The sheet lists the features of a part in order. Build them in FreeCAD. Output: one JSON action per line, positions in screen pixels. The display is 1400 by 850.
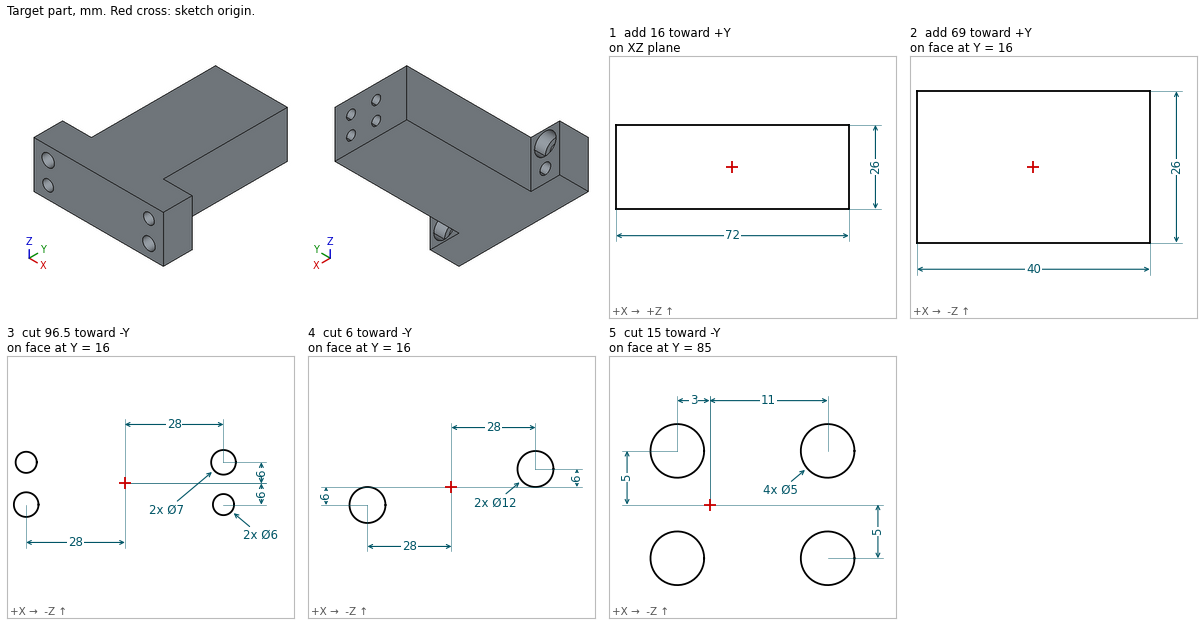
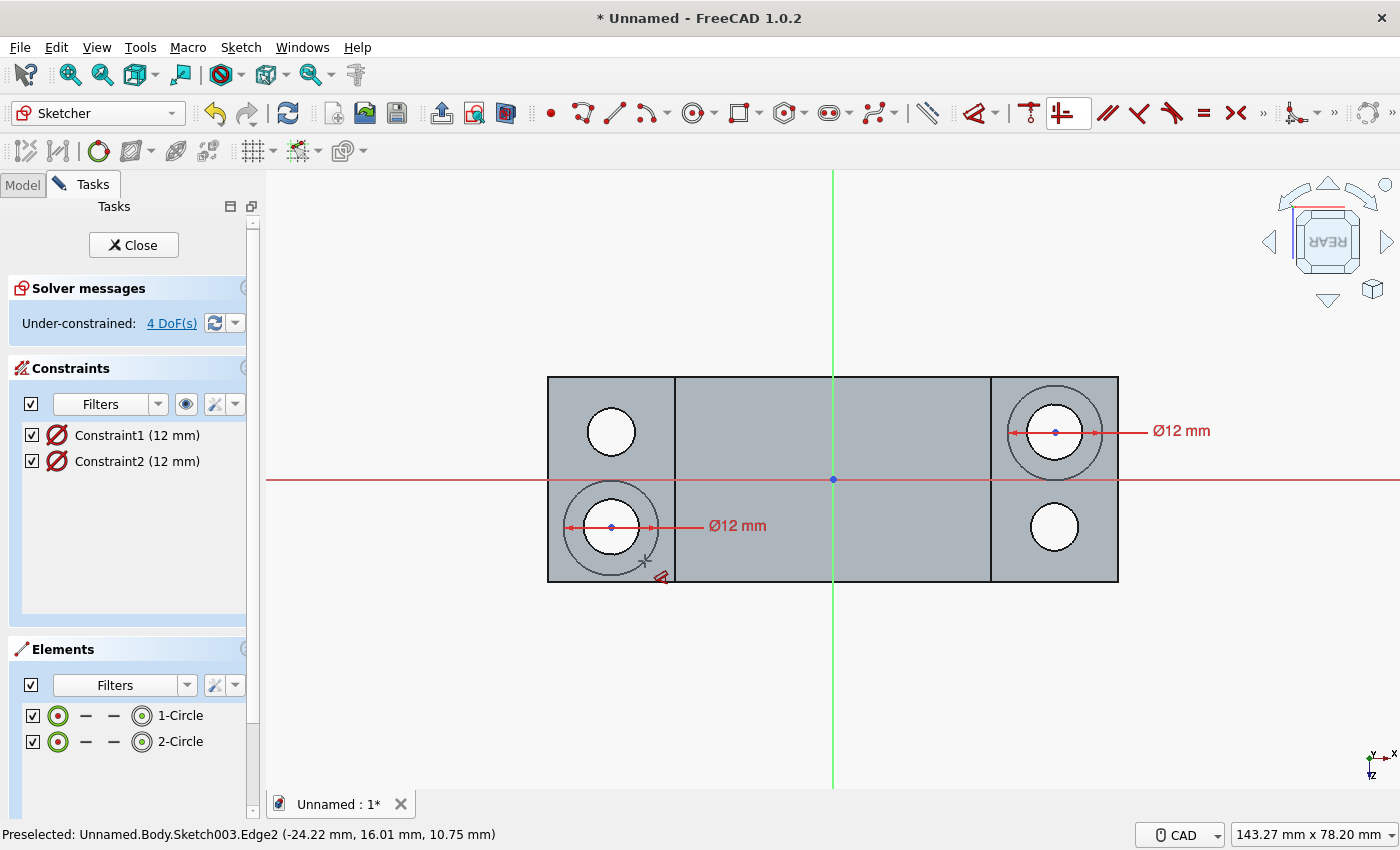
{"action": "left_click", "coordinate": [1055, 433]}
{"action": "left_click", "coordinate": [799, 456]}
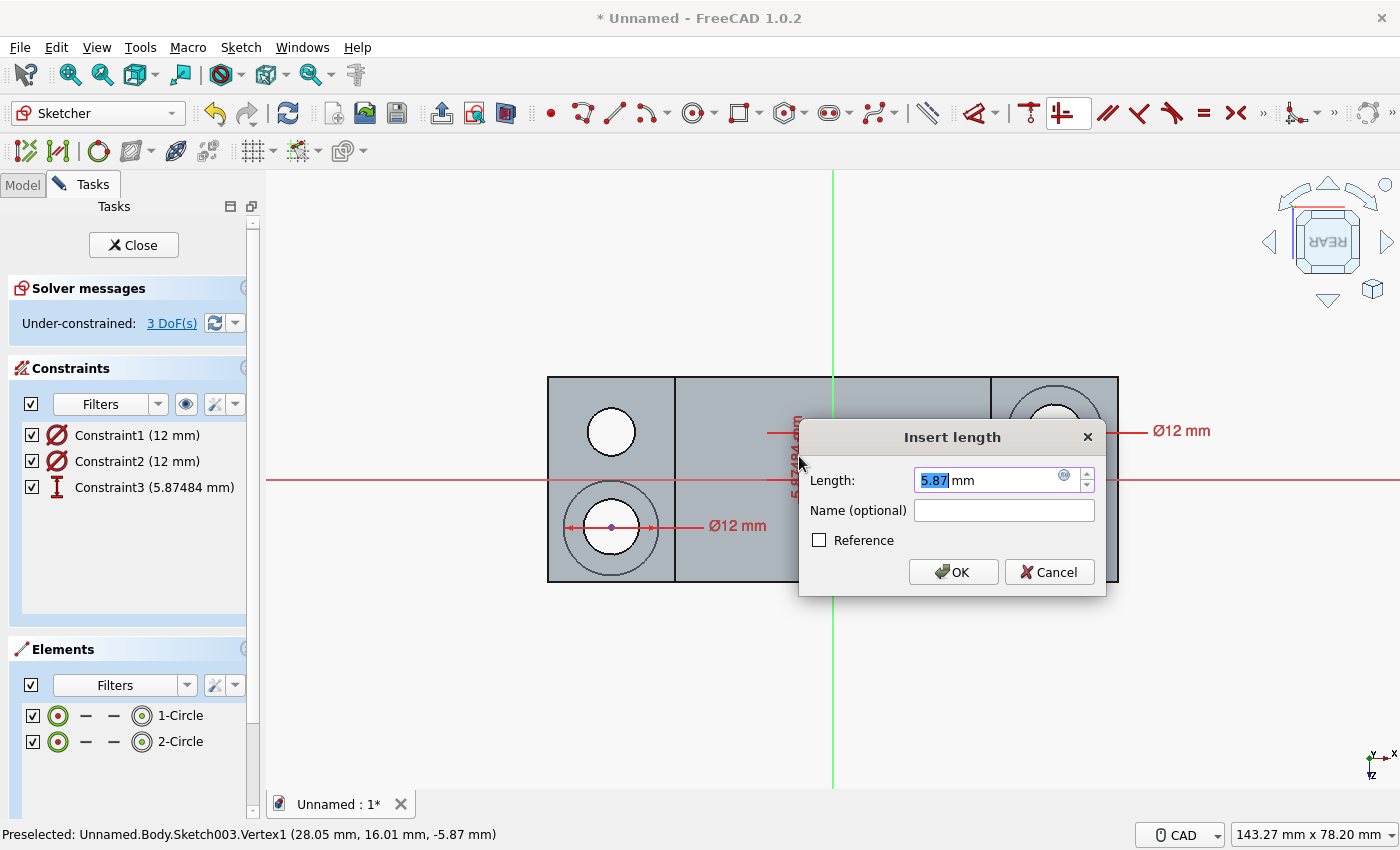
{"action": "type", "text": "6"}
{"action": "key", "text": "Return"}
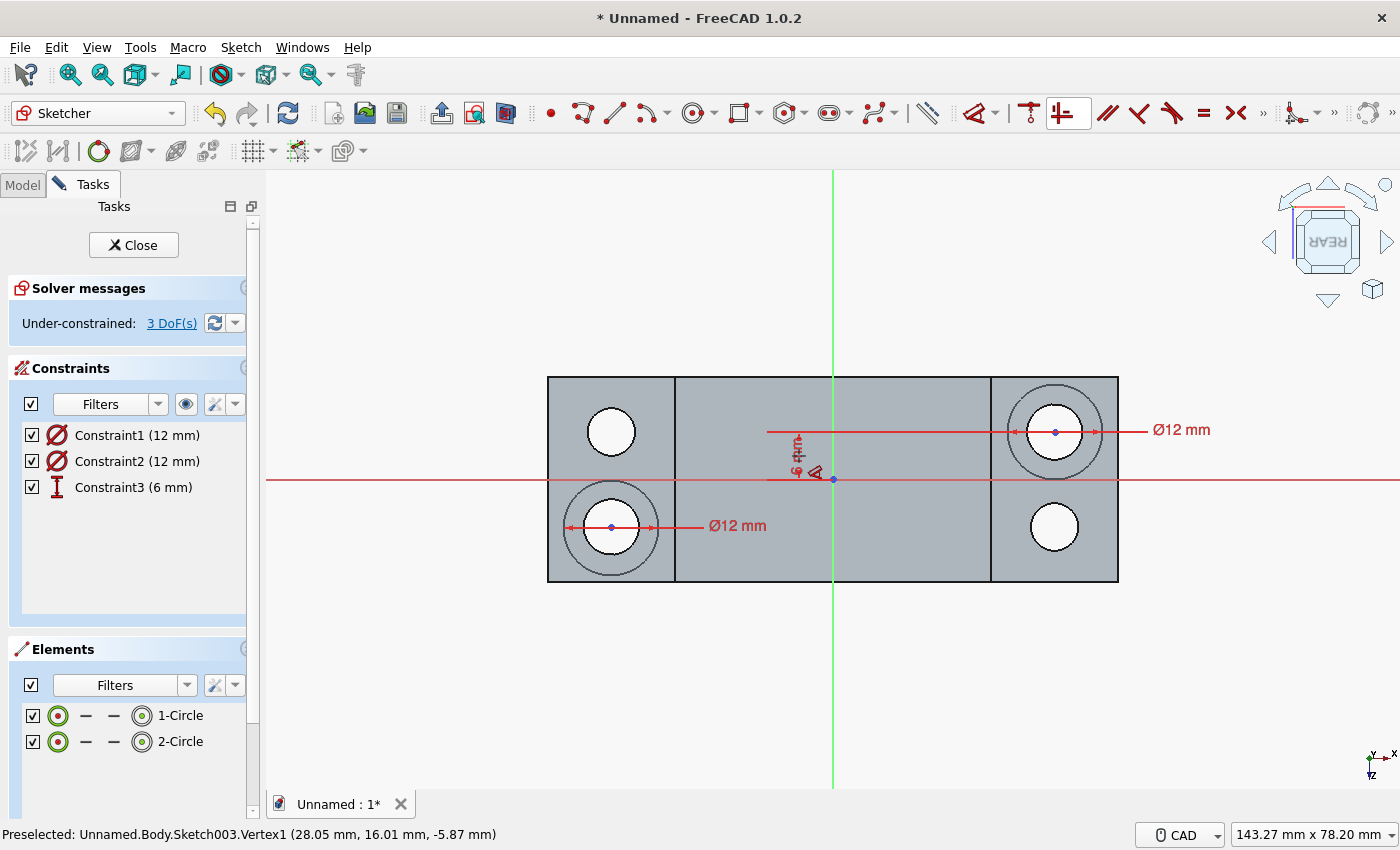
{"action": "left_click", "coordinate": [611, 528]}
{"action": "left_click", "coordinate": [867, 504]}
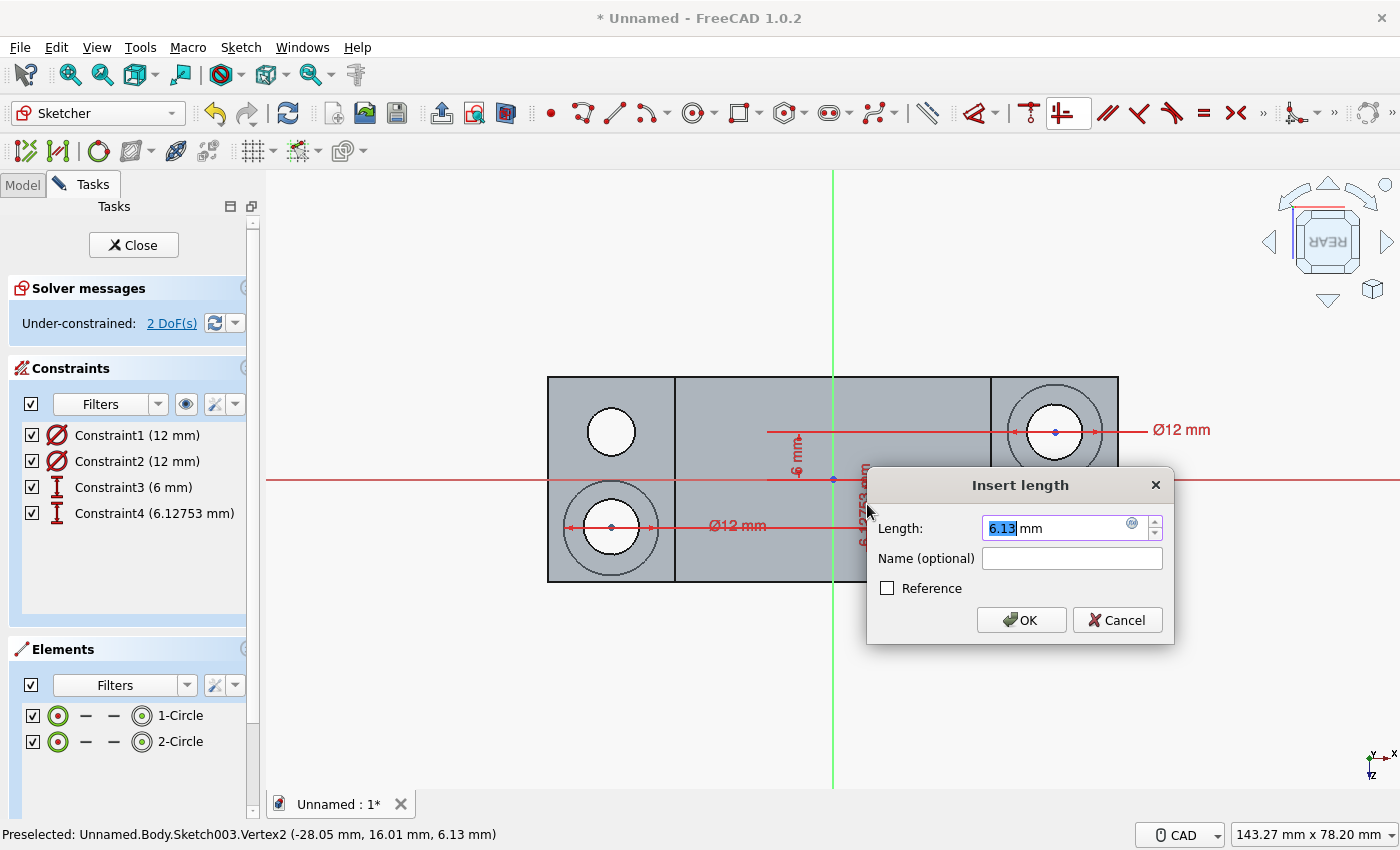
{"action": "type", "text": "6"}
{"action": "key", "text": "Return"}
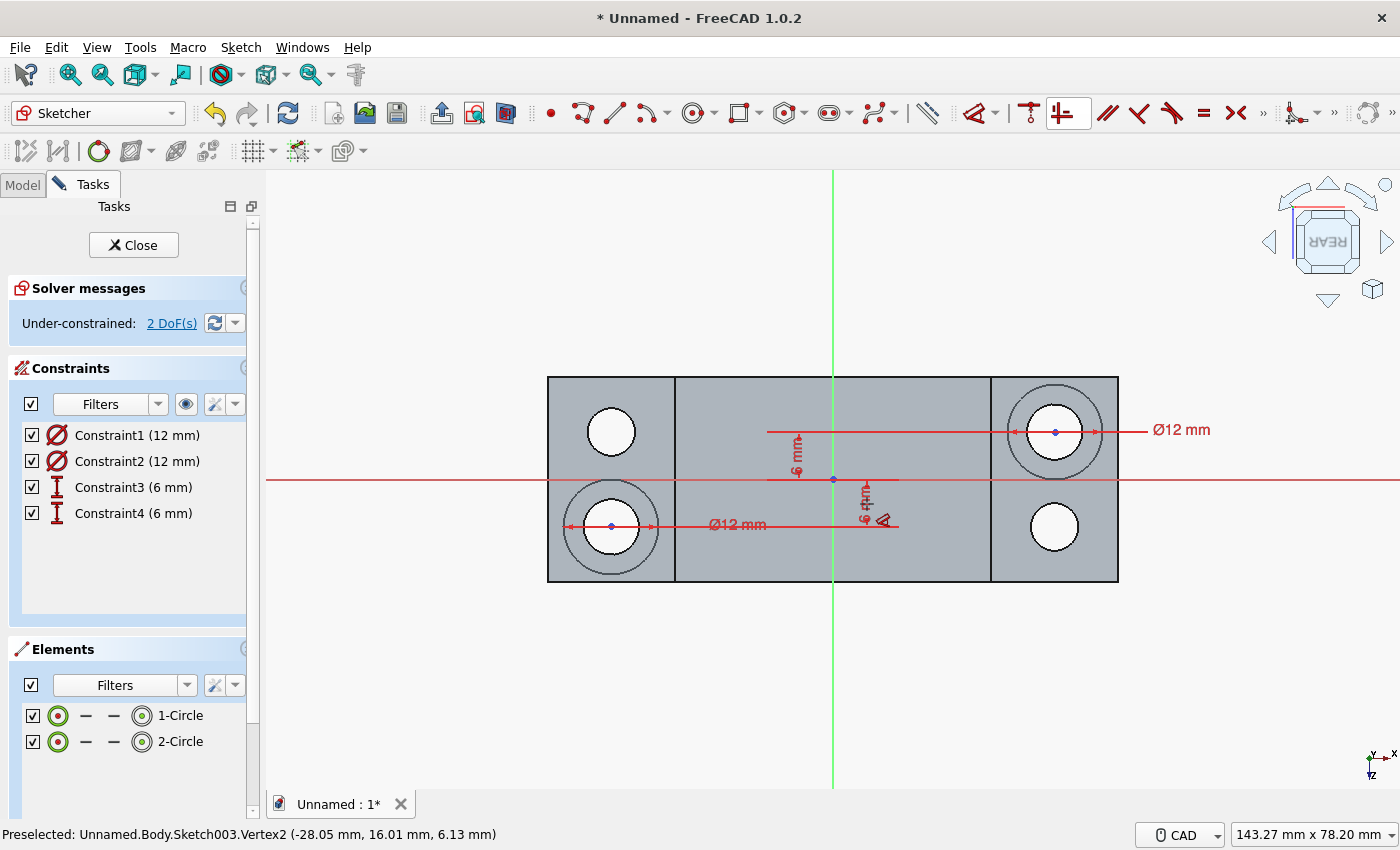
{"action": "left_click", "coordinate": [1055, 432]}
{"action": "left_click", "coordinate": [944, 398]}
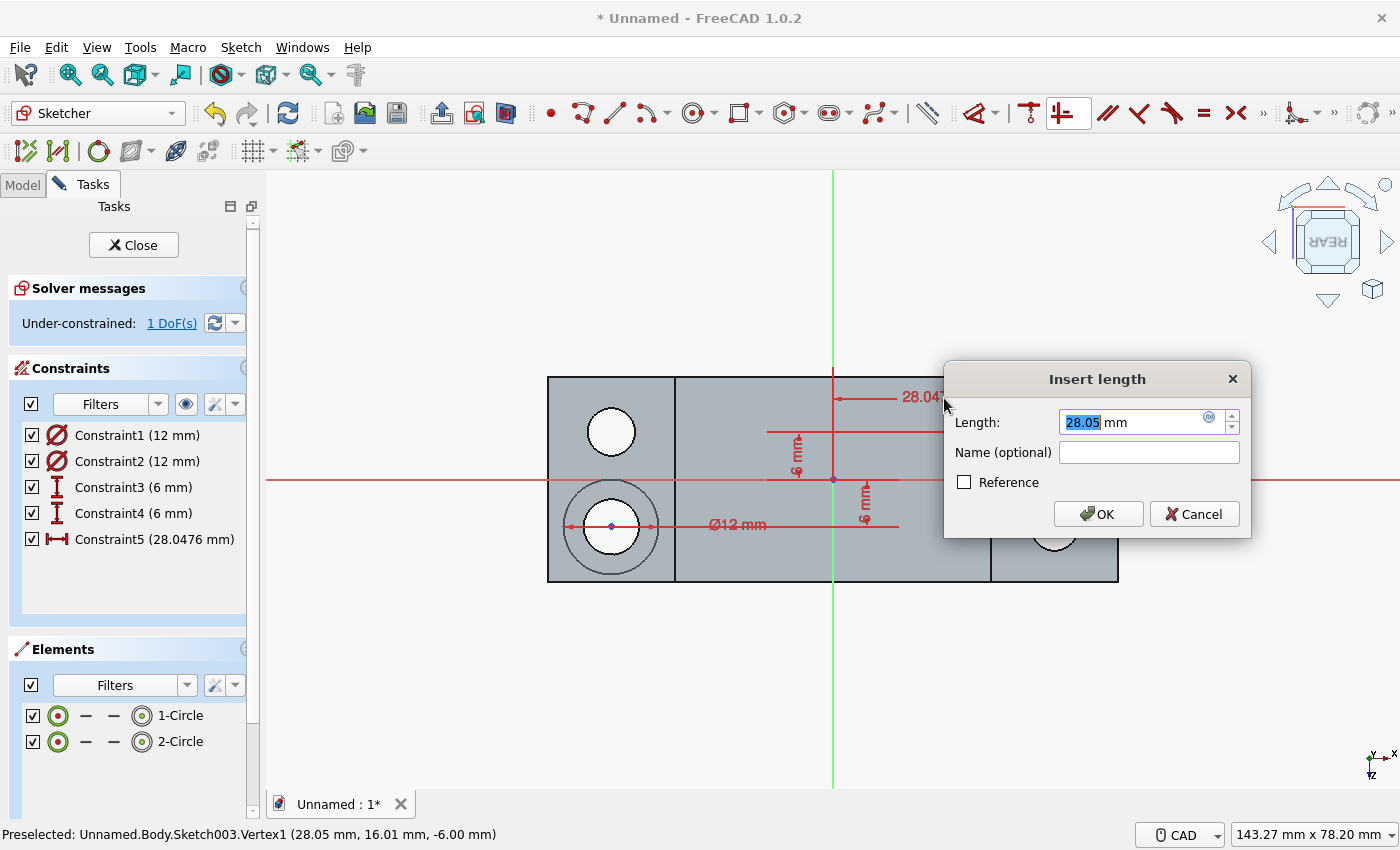
{"action": "type", "text": "28"}
{"action": "key", "text": "Return"}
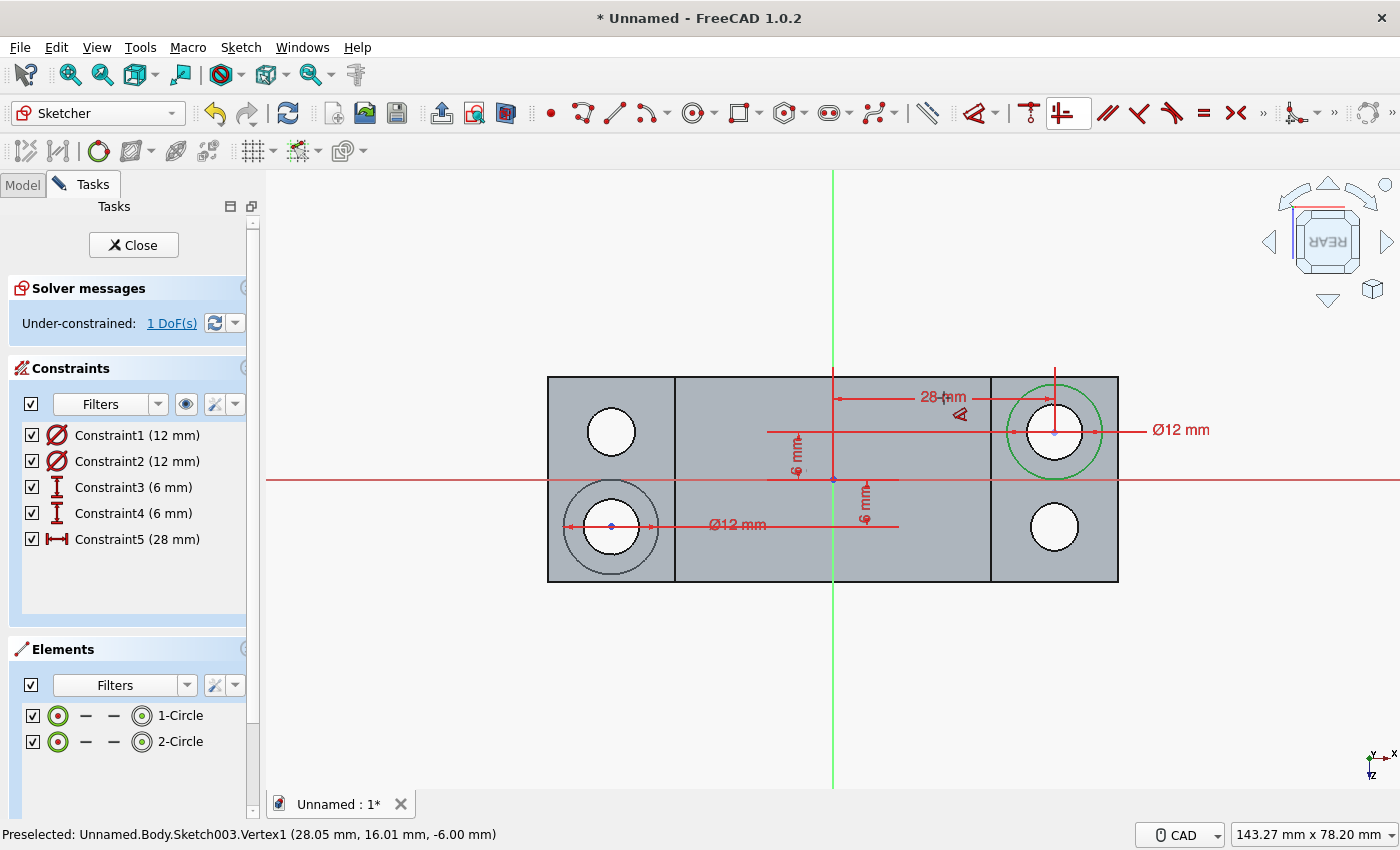
{"action": "left_click", "coordinate": [611, 527]}
{"action": "left_click", "coordinate": [722, 561]}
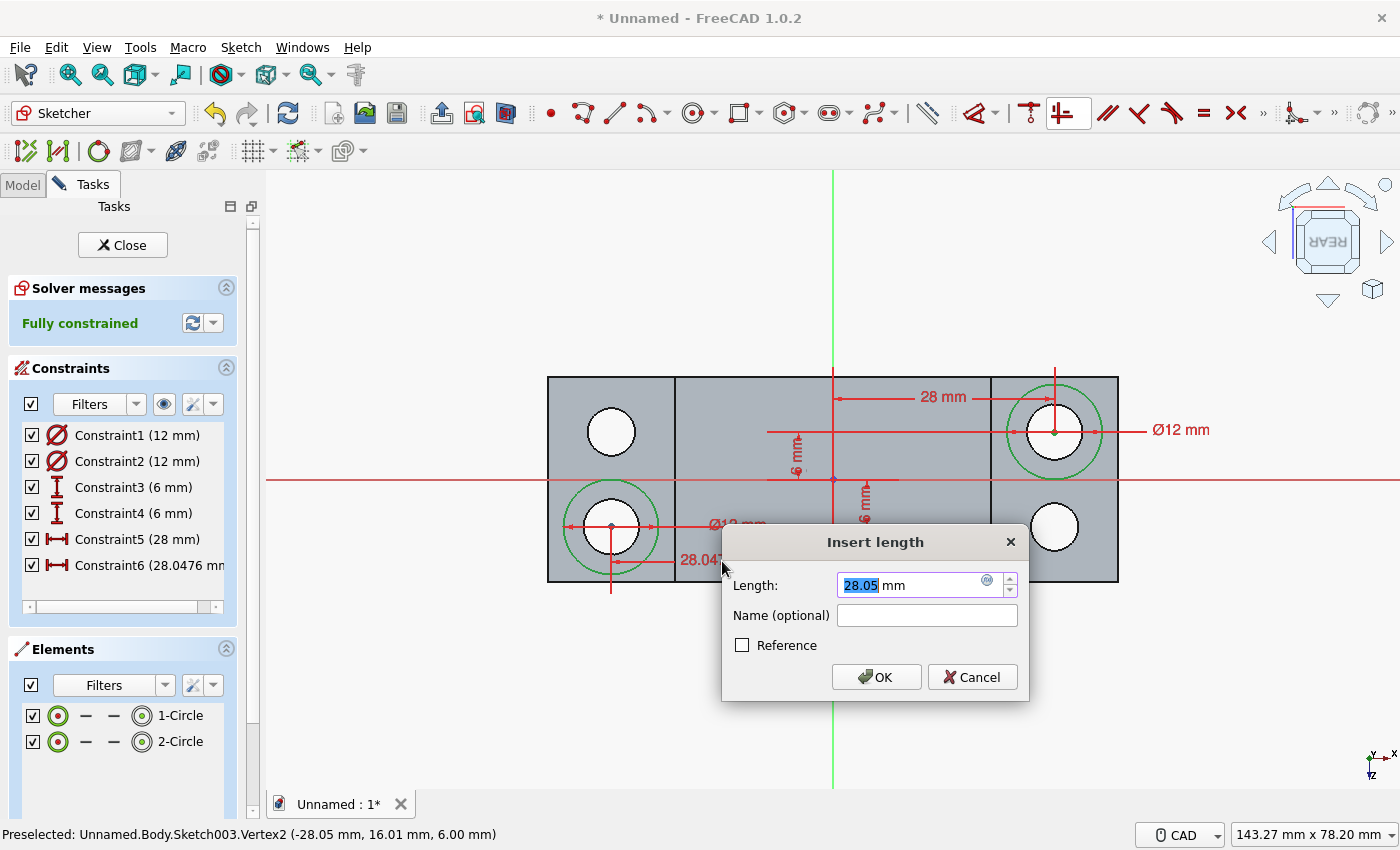
{"action": "type", "text": "28"}
{"action": "key", "text": "Return"}
{"action": "key", "text": "Escape"}